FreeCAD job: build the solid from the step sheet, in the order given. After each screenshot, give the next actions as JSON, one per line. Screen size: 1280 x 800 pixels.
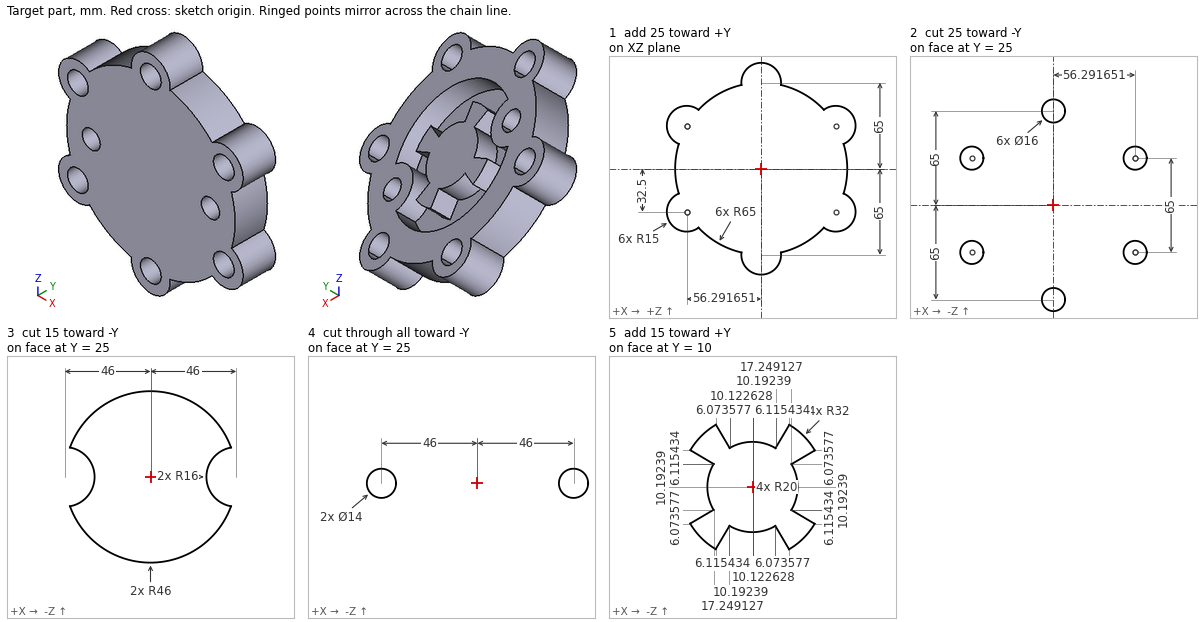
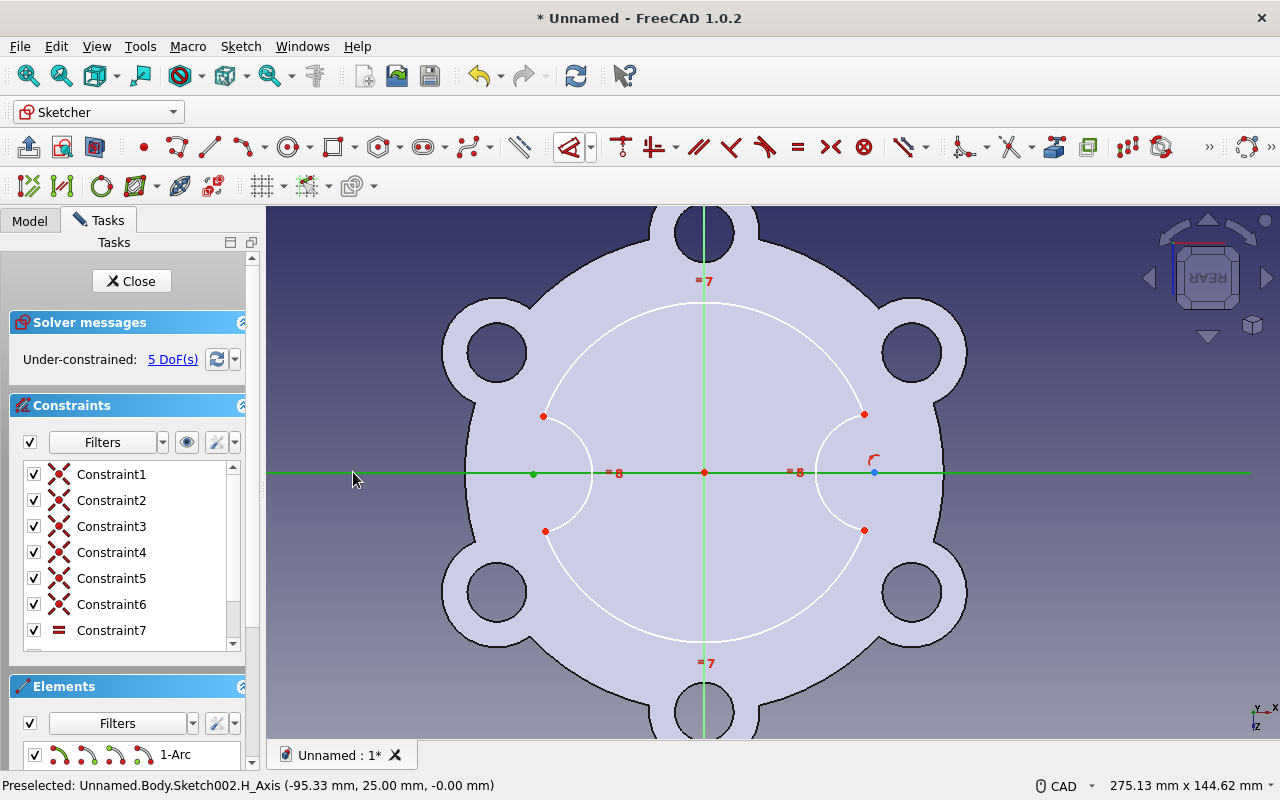
{"action": "left_click", "coordinate": [621, 148]}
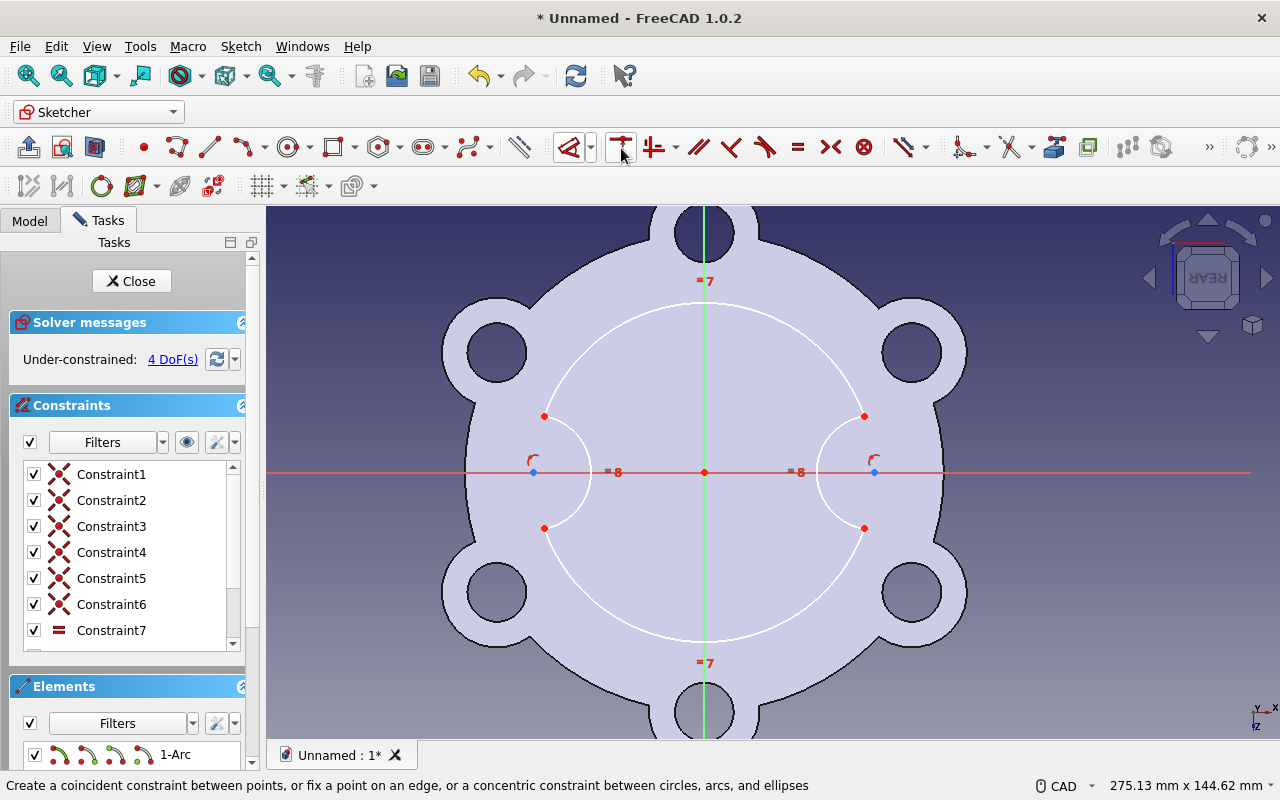
{"action": "left_click", "coordinate": [624, 622]}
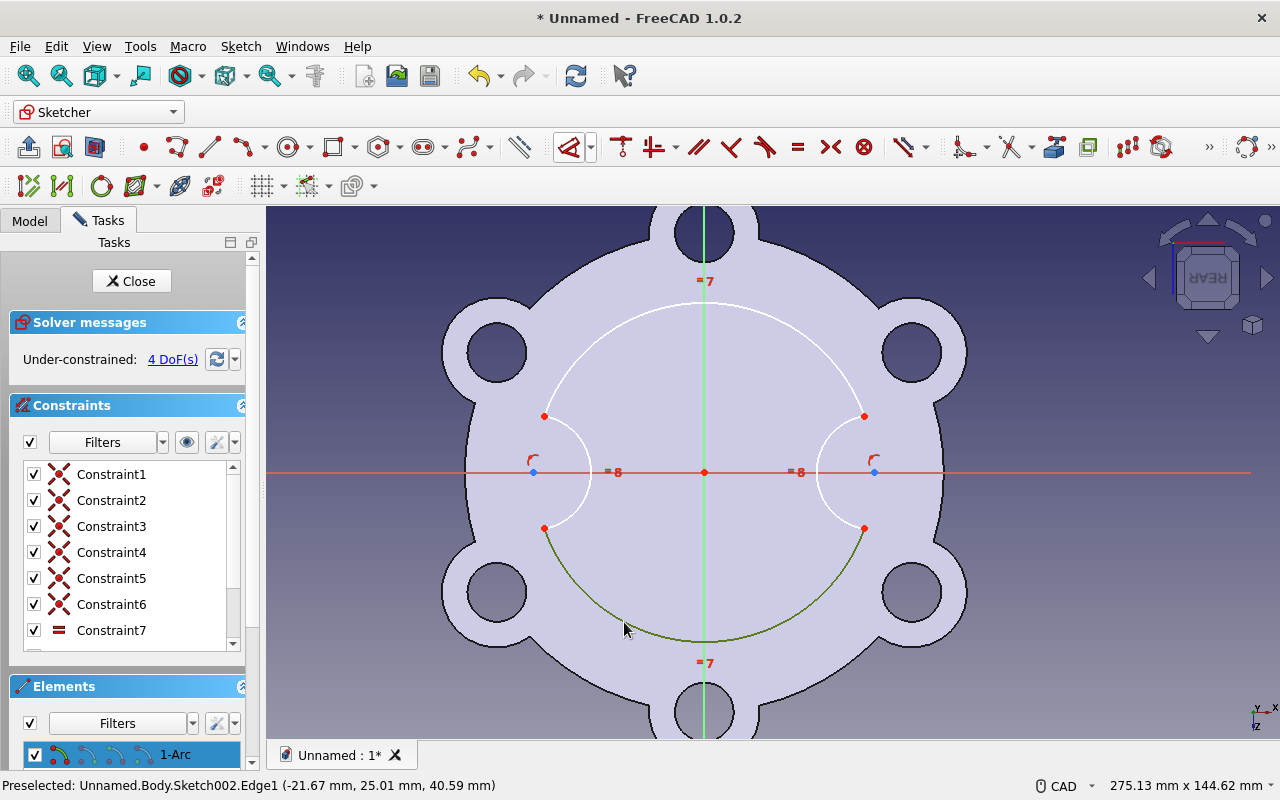
{"action": "key", "text": "k r"}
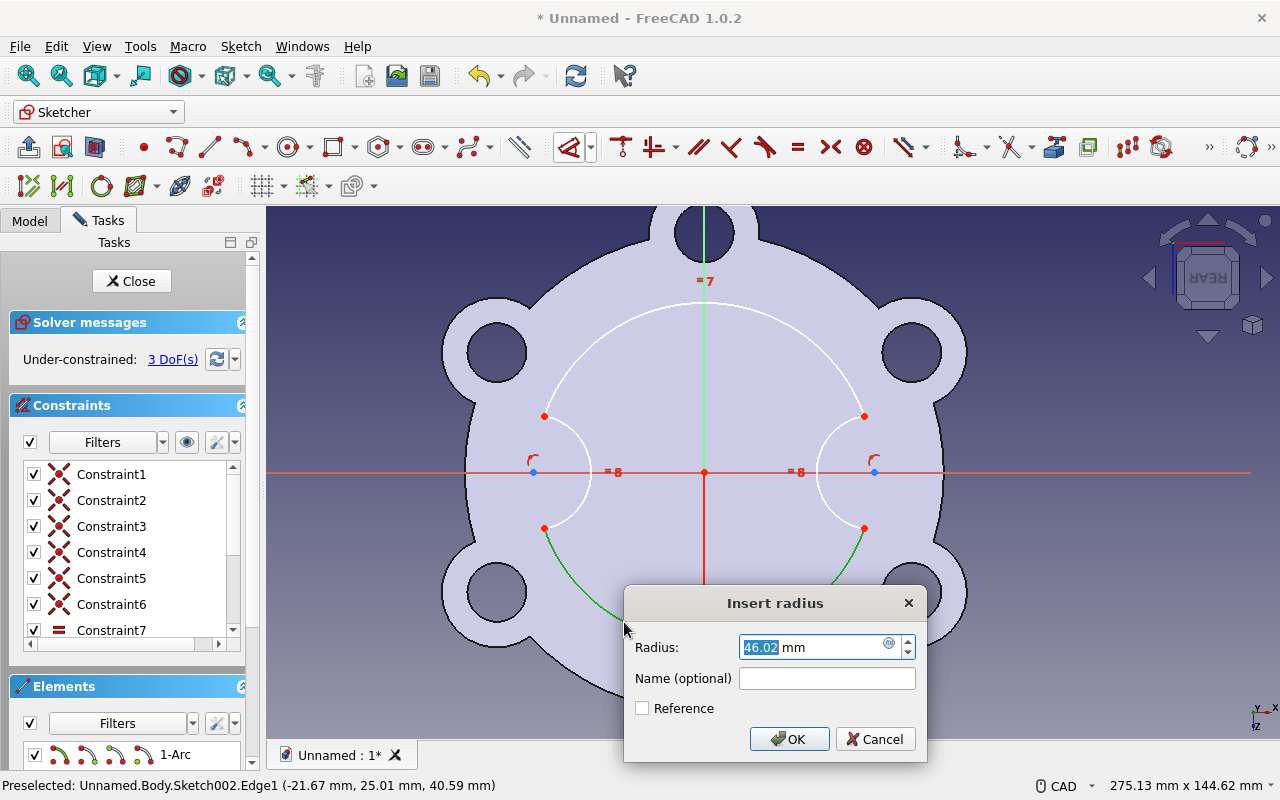
{"action": "type", "text": "46"}
{"action": "key", "text": "Return"}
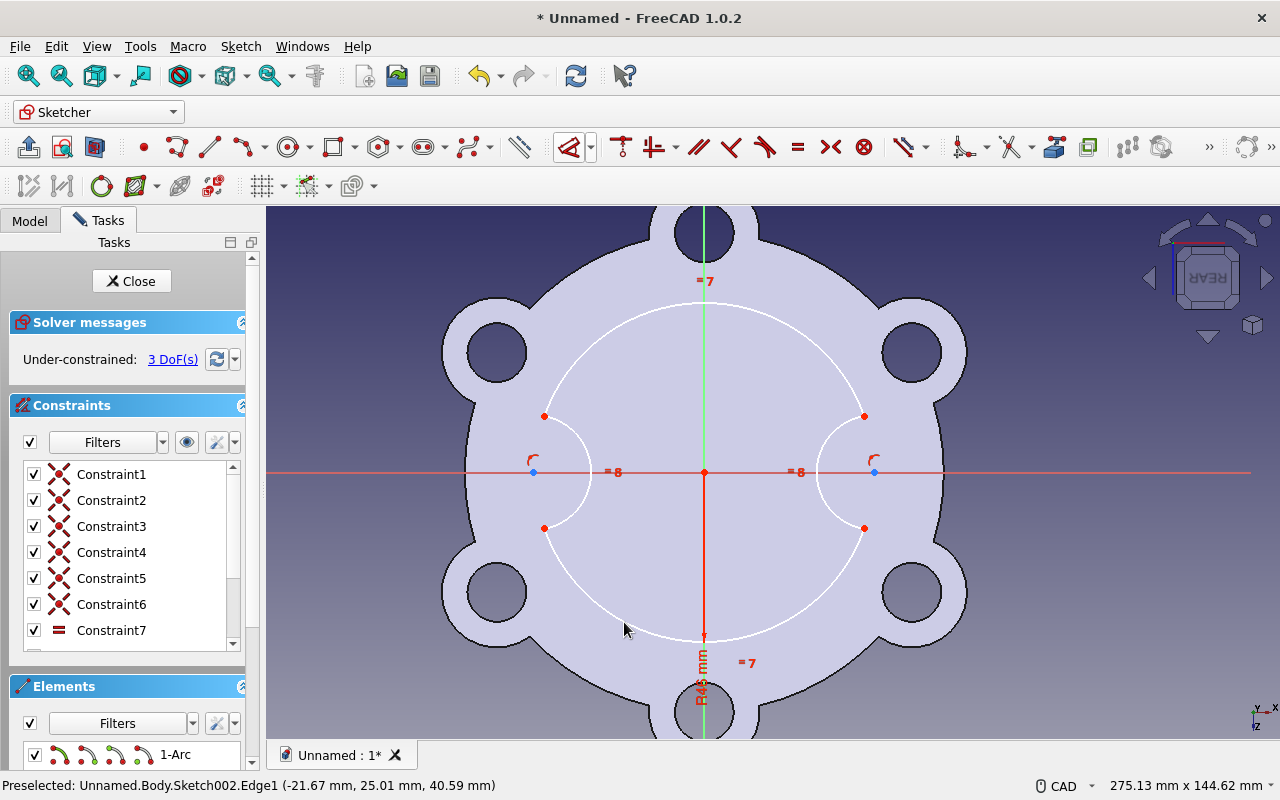
{"action": "left_click", "coordinate": [825, 442]}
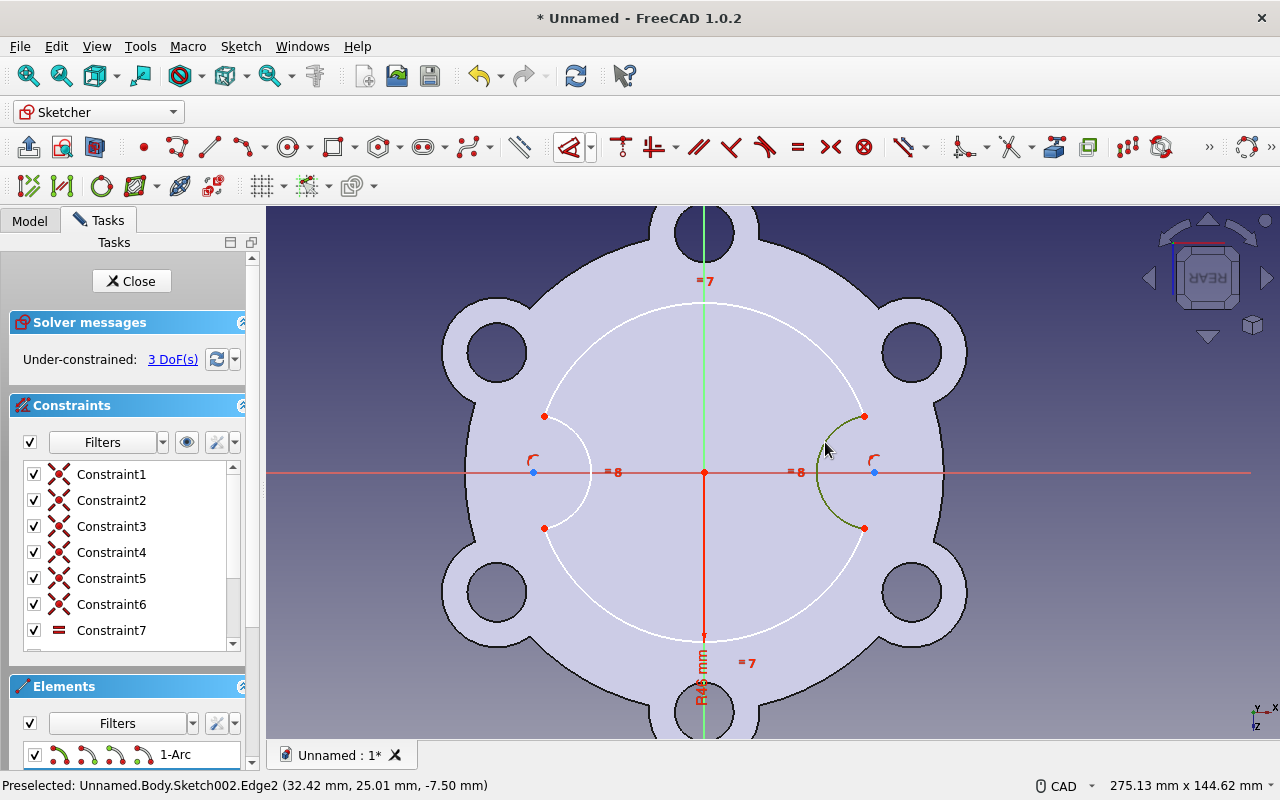
{"action": "key", "text": "k r"}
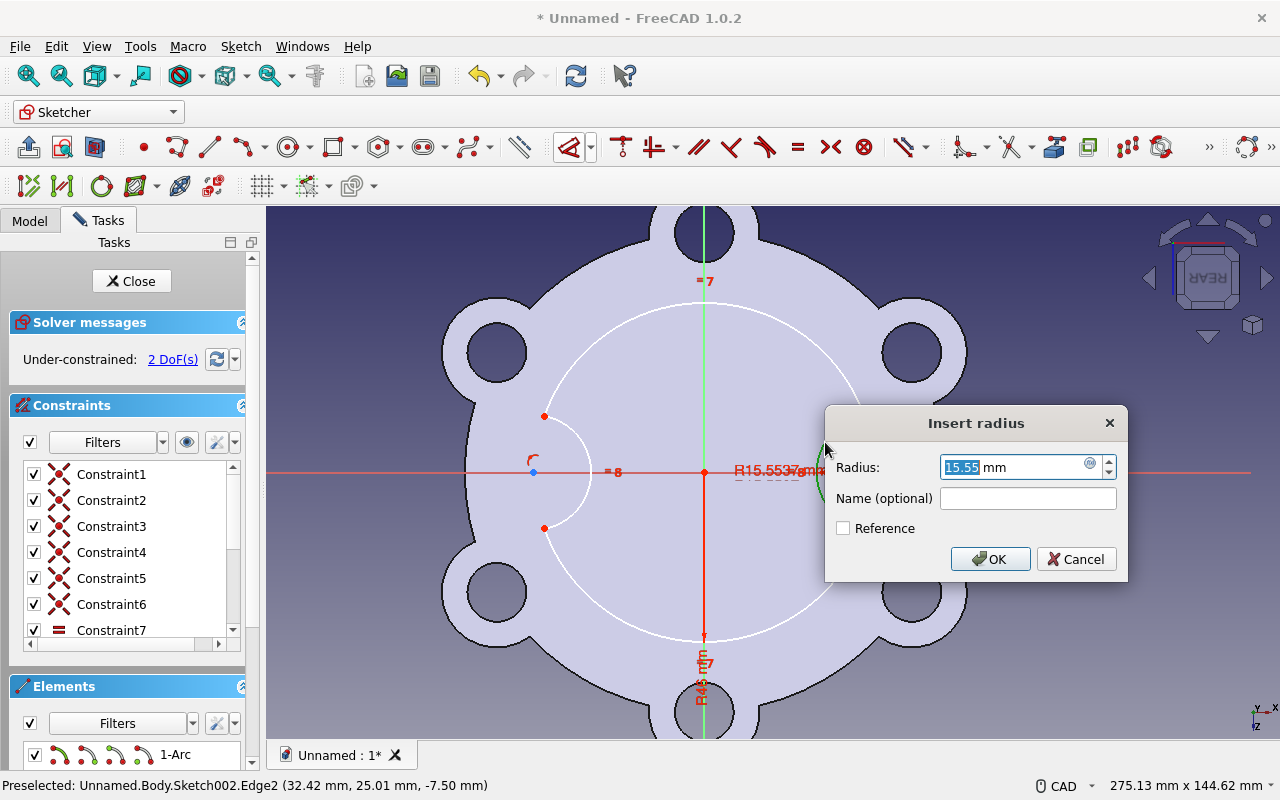
{"action": "type", "text": "16"}
{"action": "key", "text": "Return"}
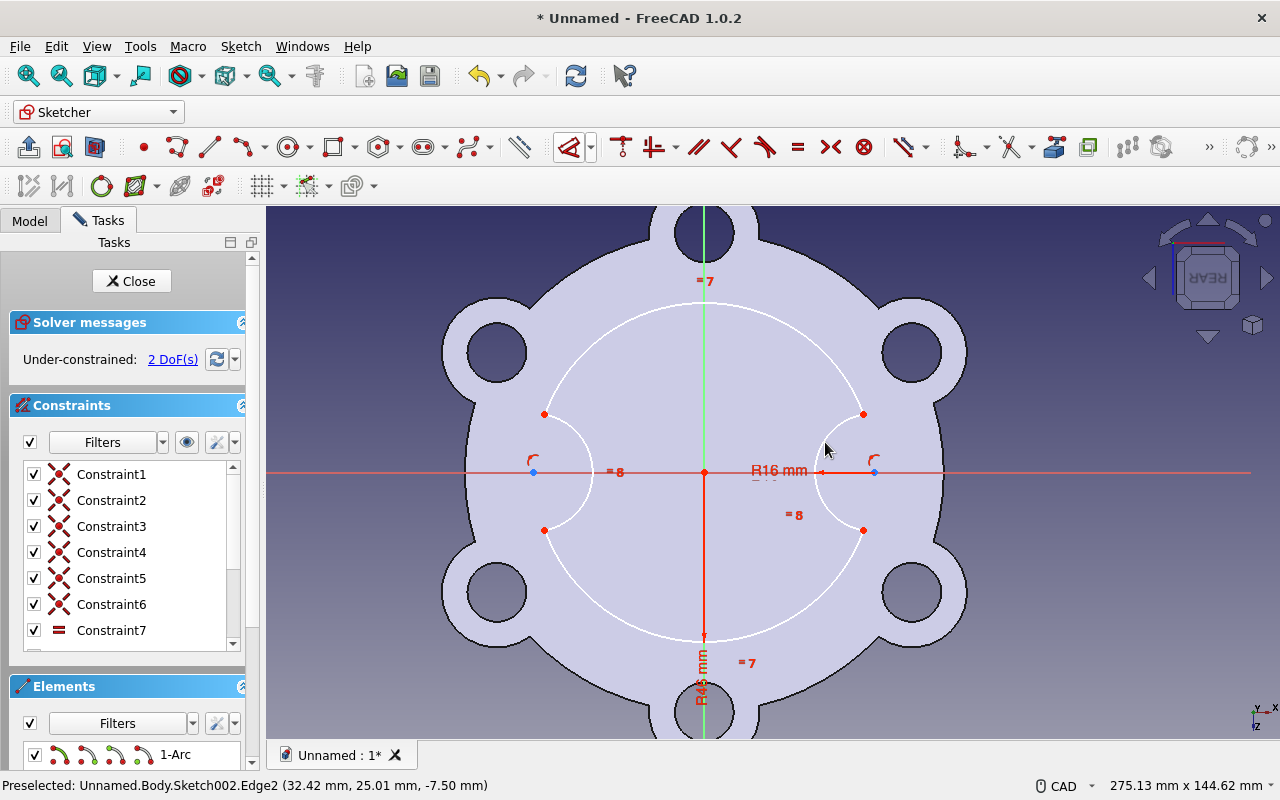
{"action": "left_click", "coordinate": [874, 472]}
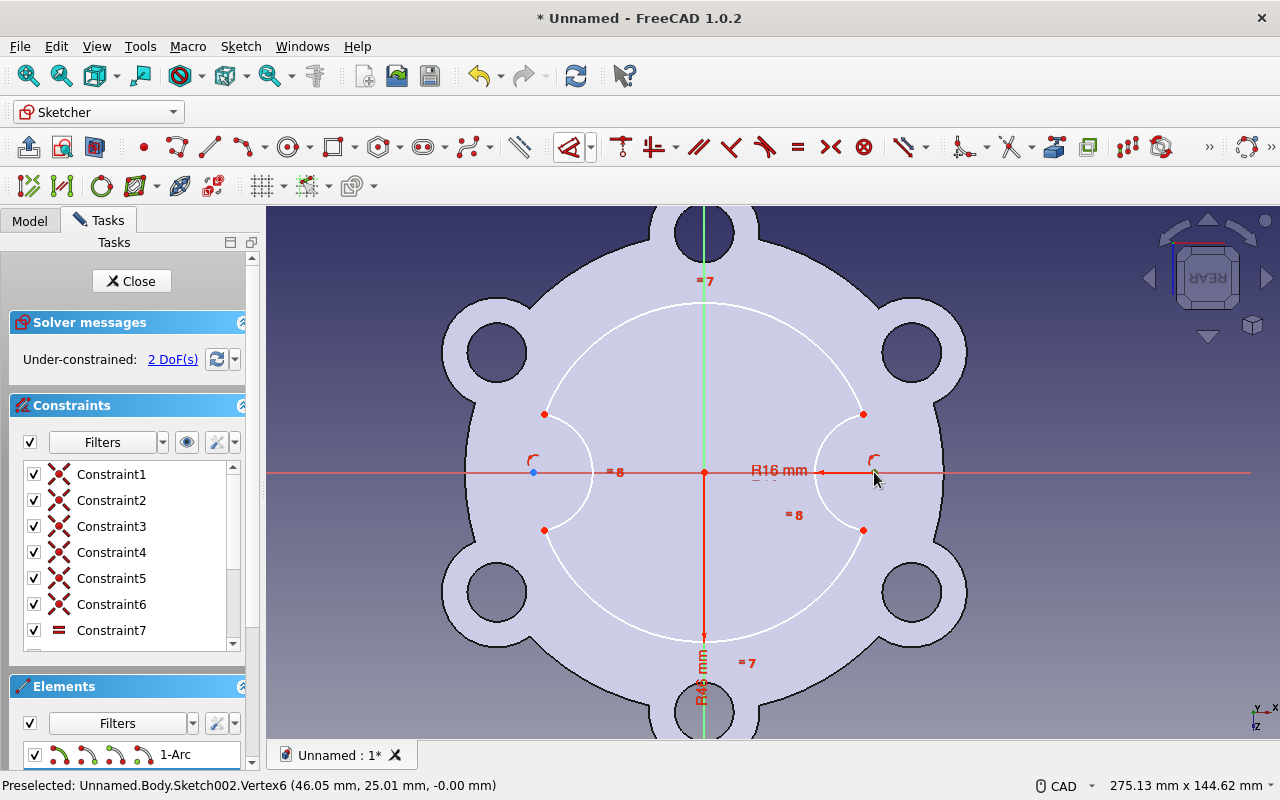
{"action": "left_click", "coordinate": [590, 148]}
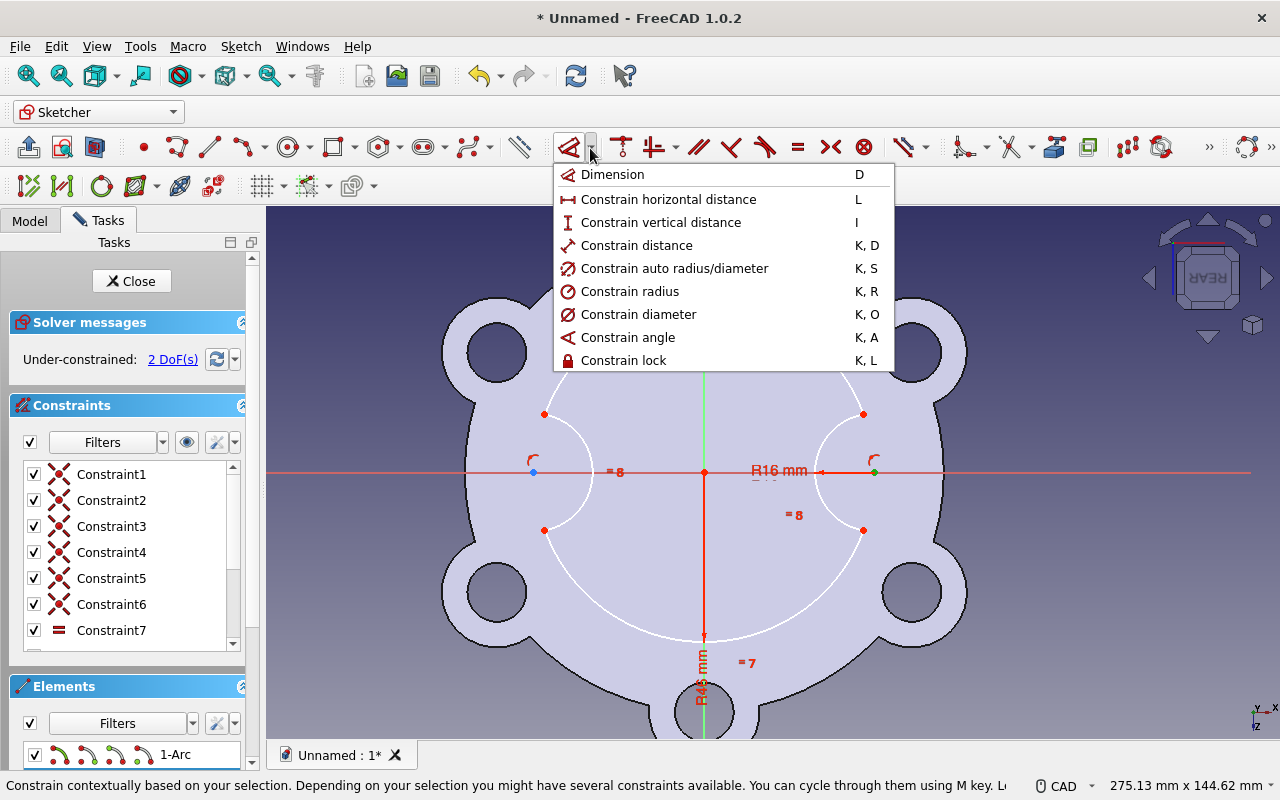
{"action": "left_click", "coordinate": [724, 200]}